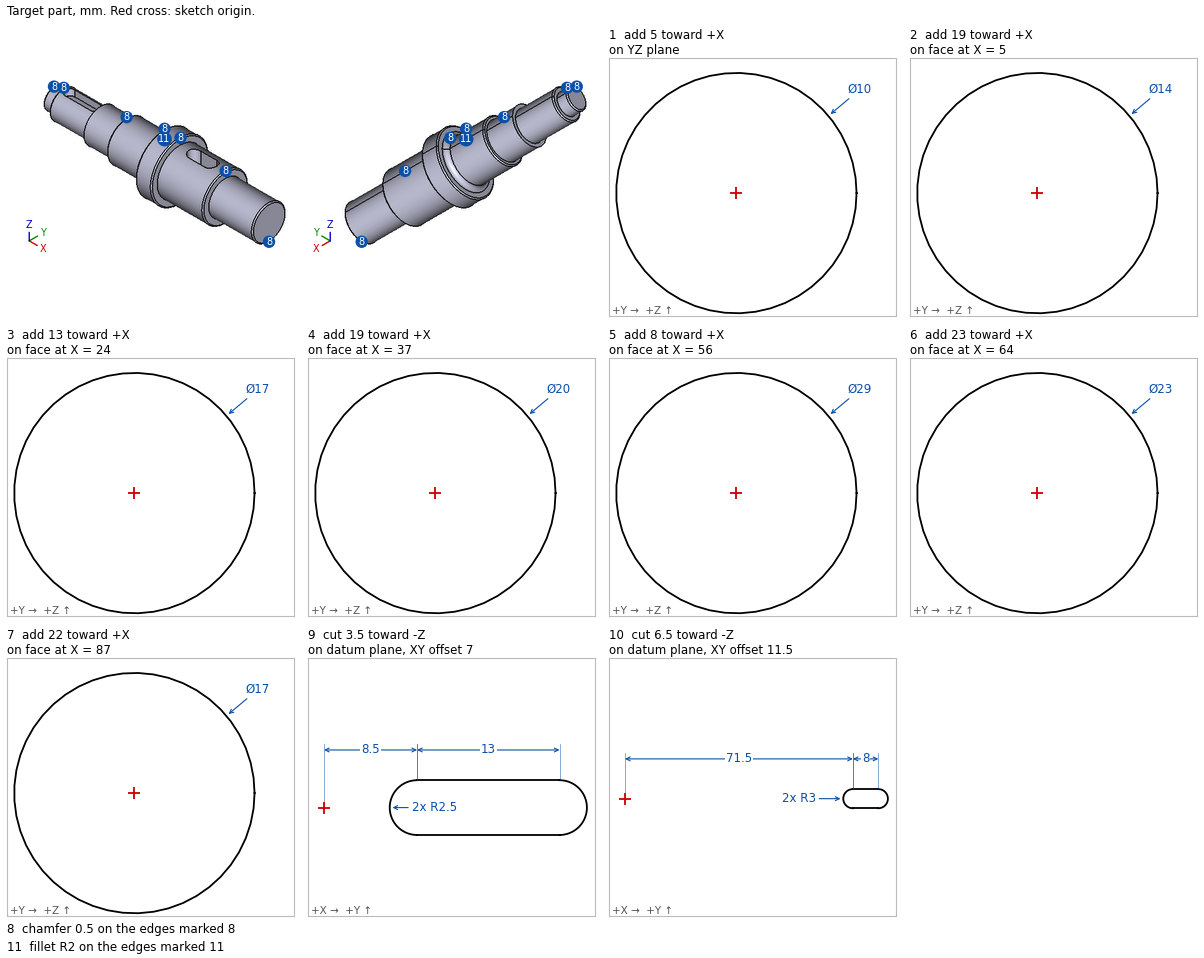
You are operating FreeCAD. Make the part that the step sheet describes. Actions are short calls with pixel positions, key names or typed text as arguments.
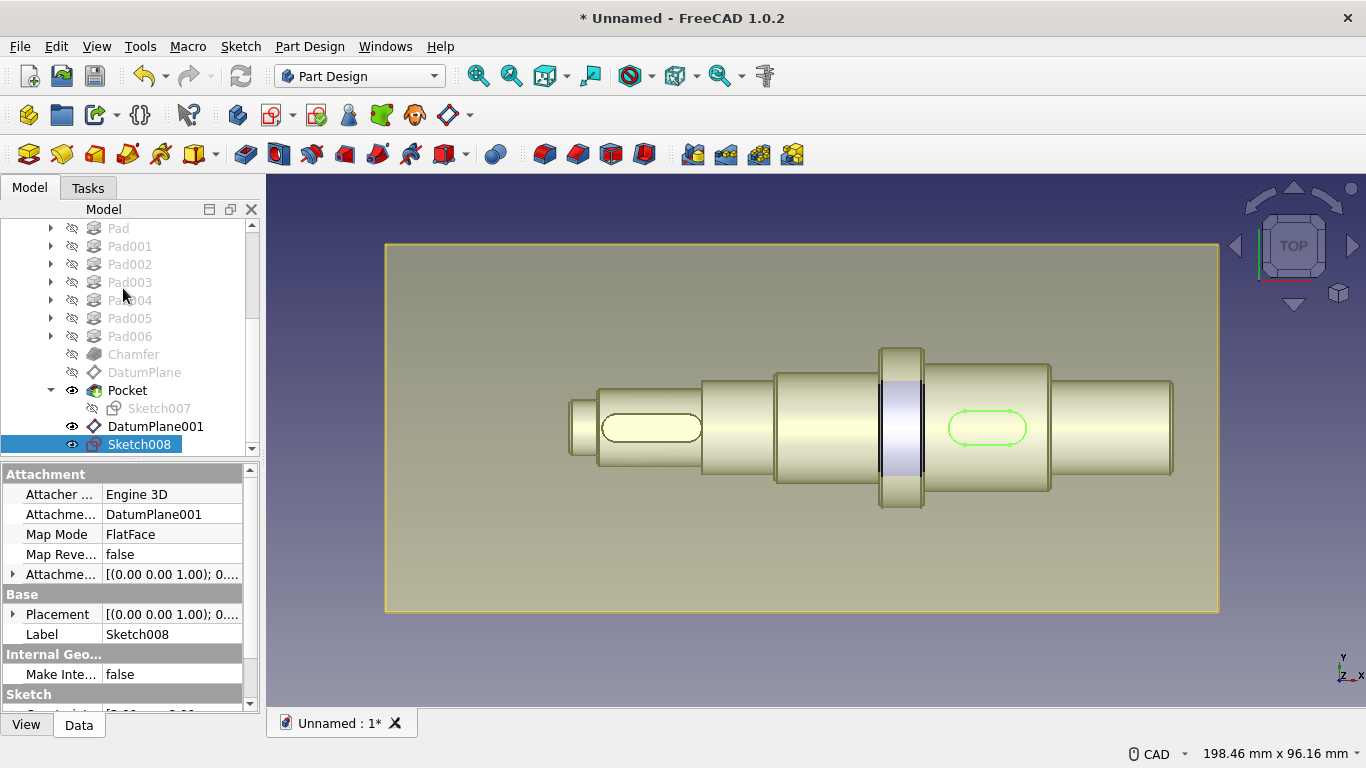
click(246, 154)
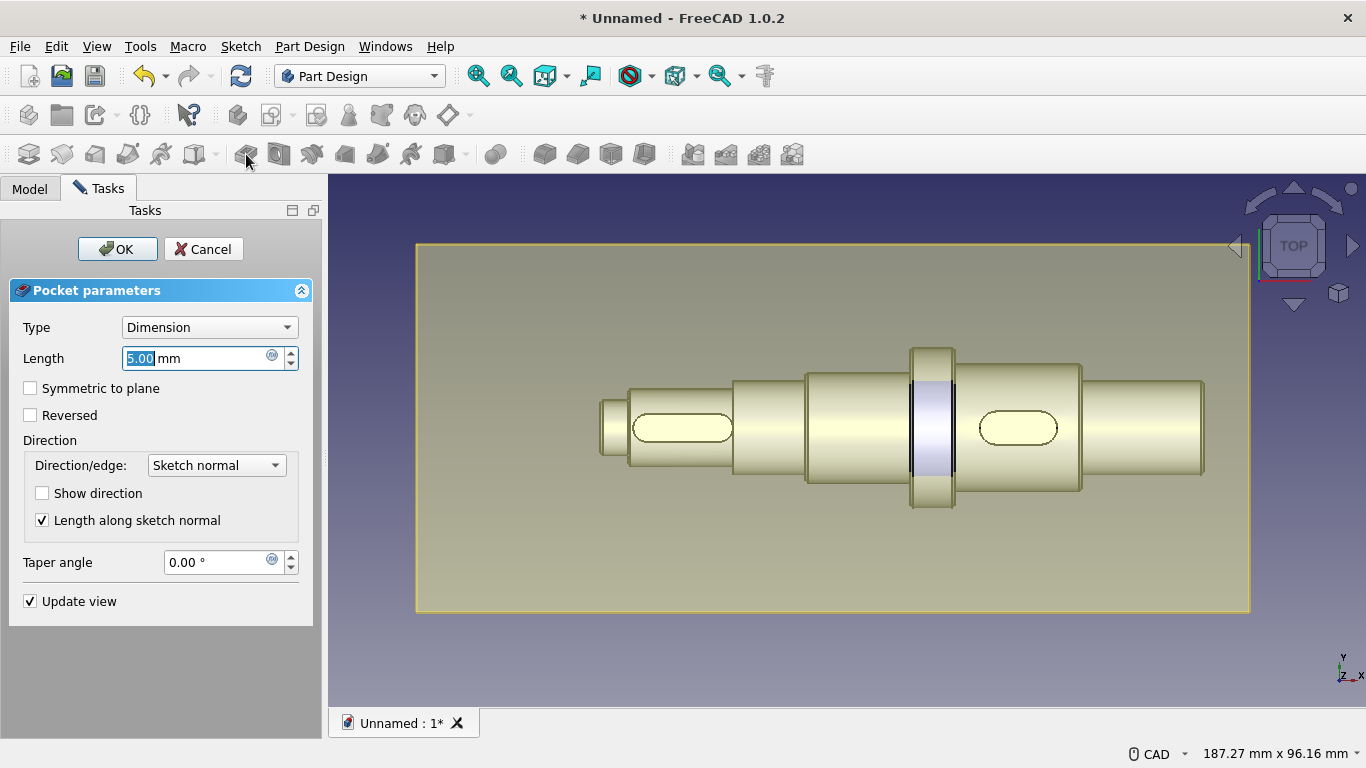
text(6.5)
key(Tab)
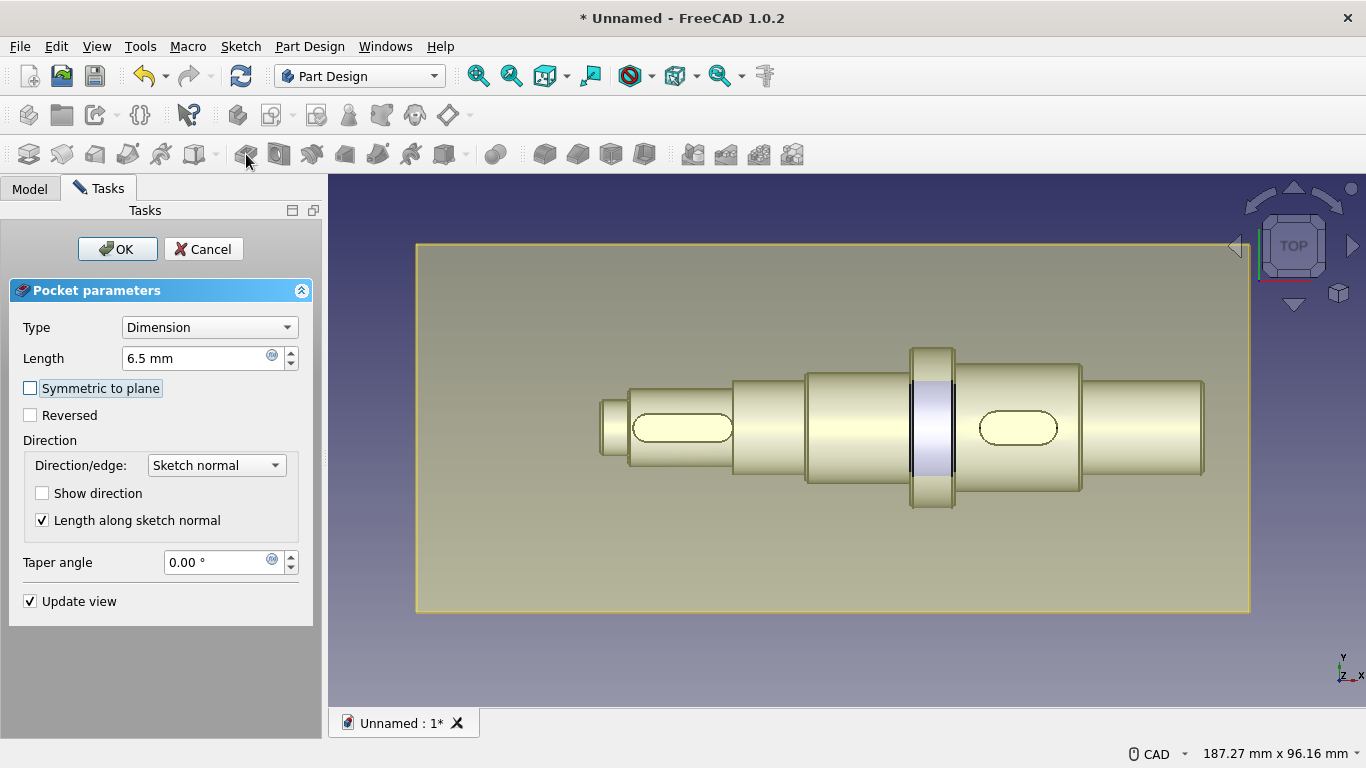
click(118, 249)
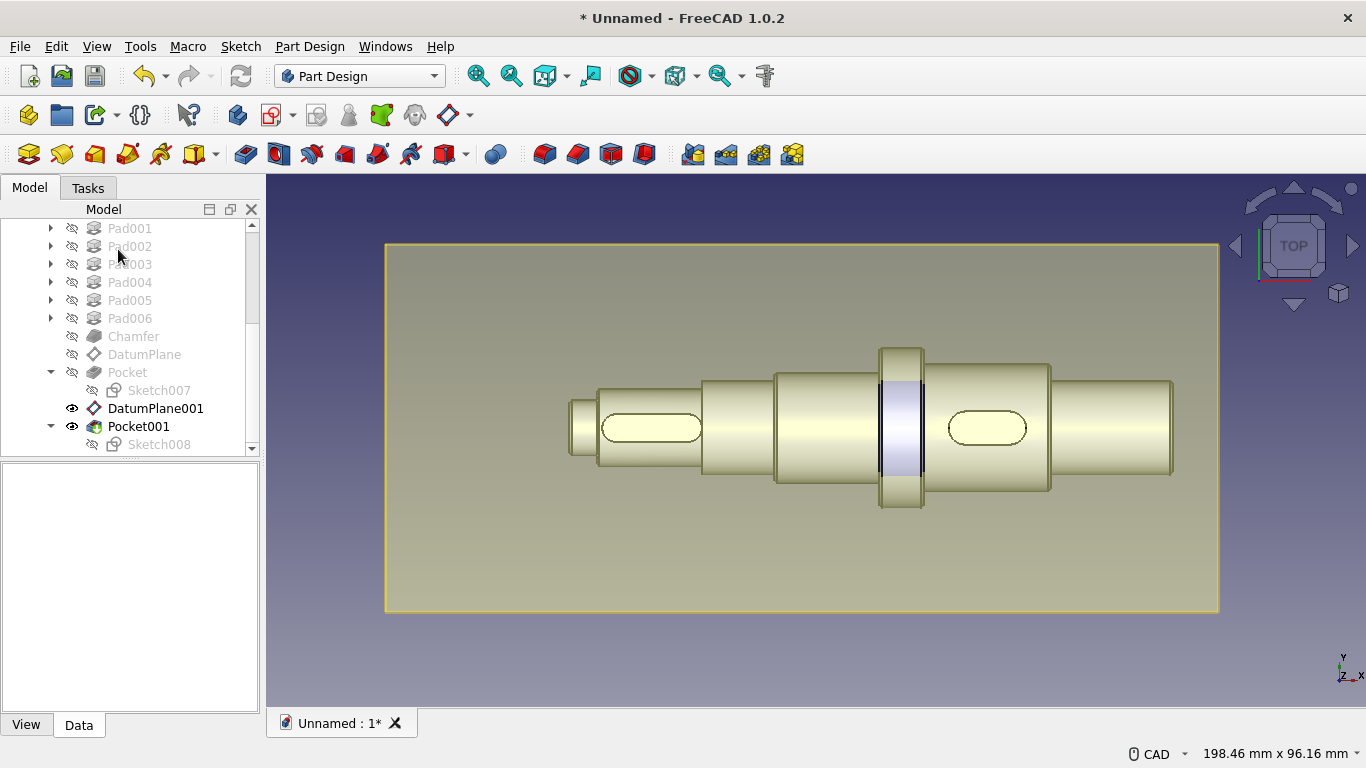
click(117, 408)
key(space)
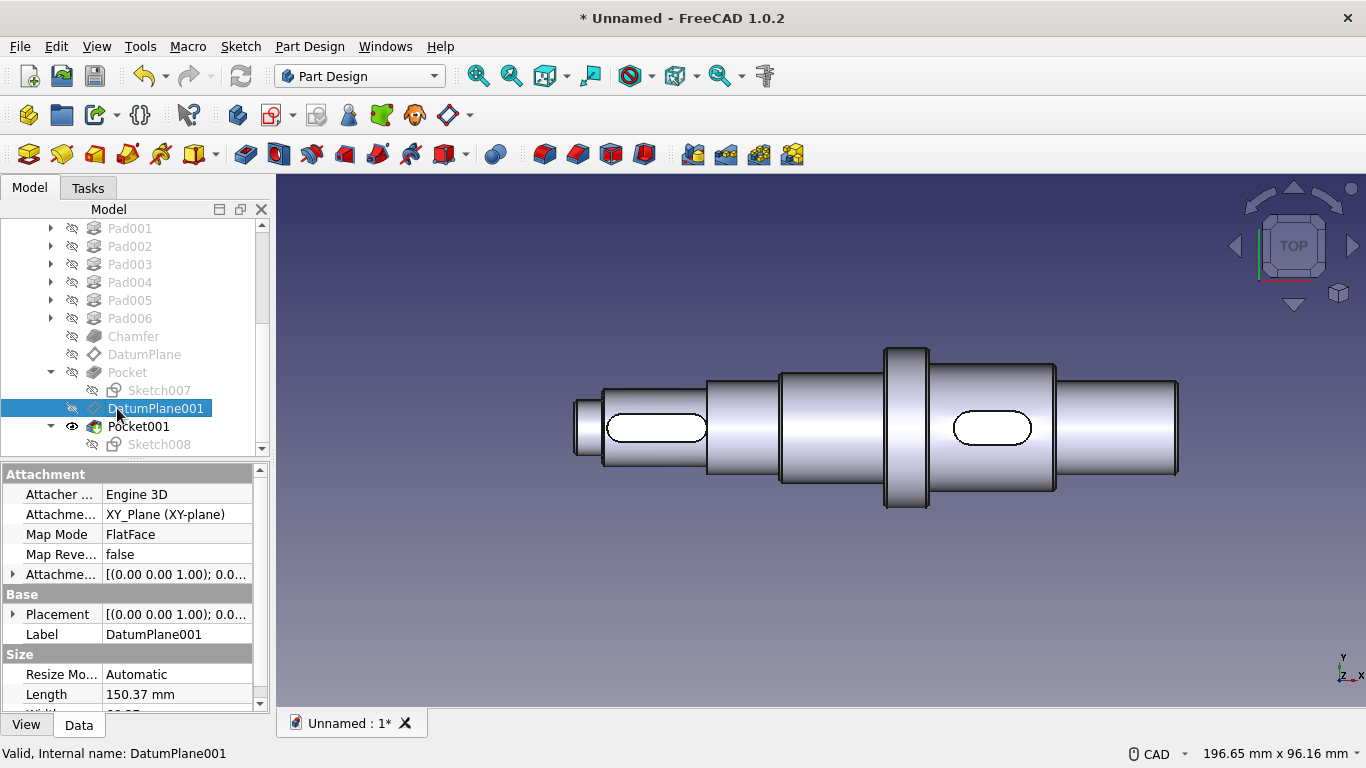
key(0)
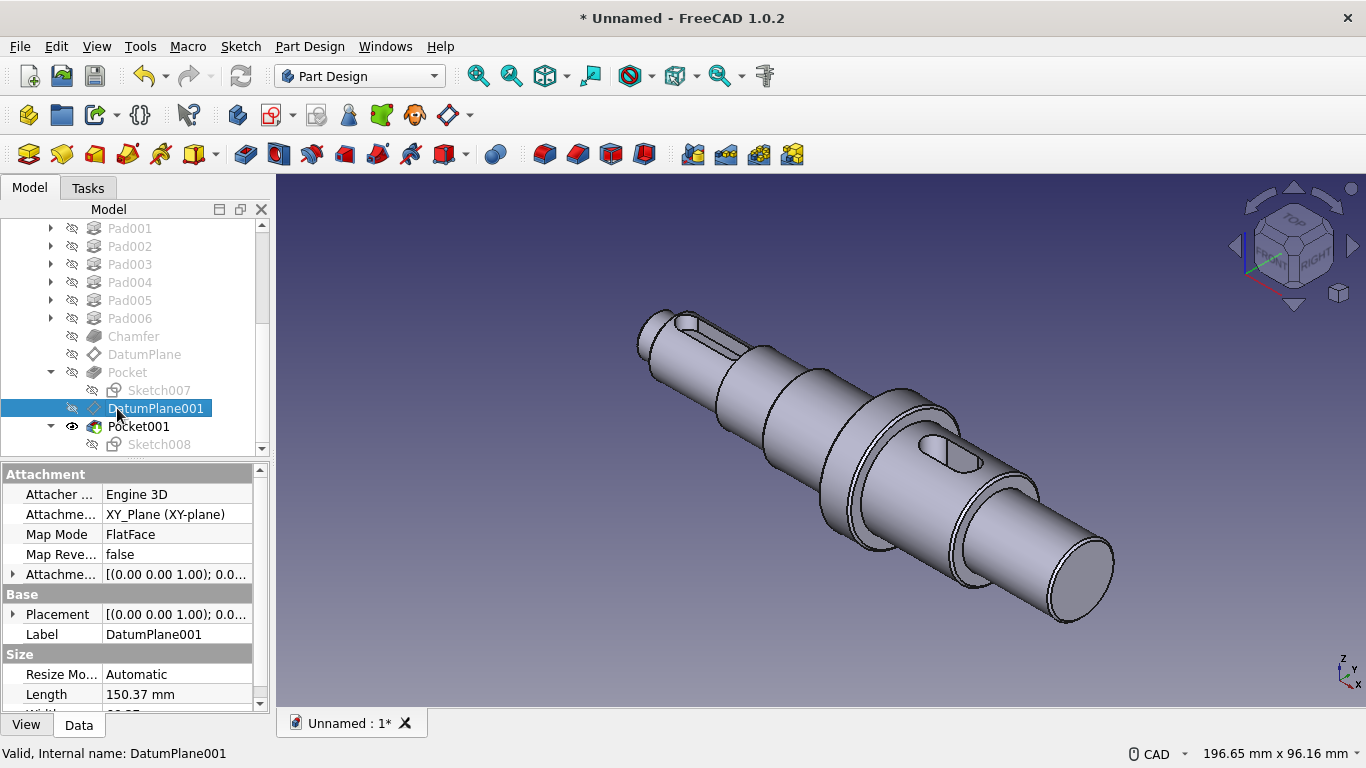
key(2)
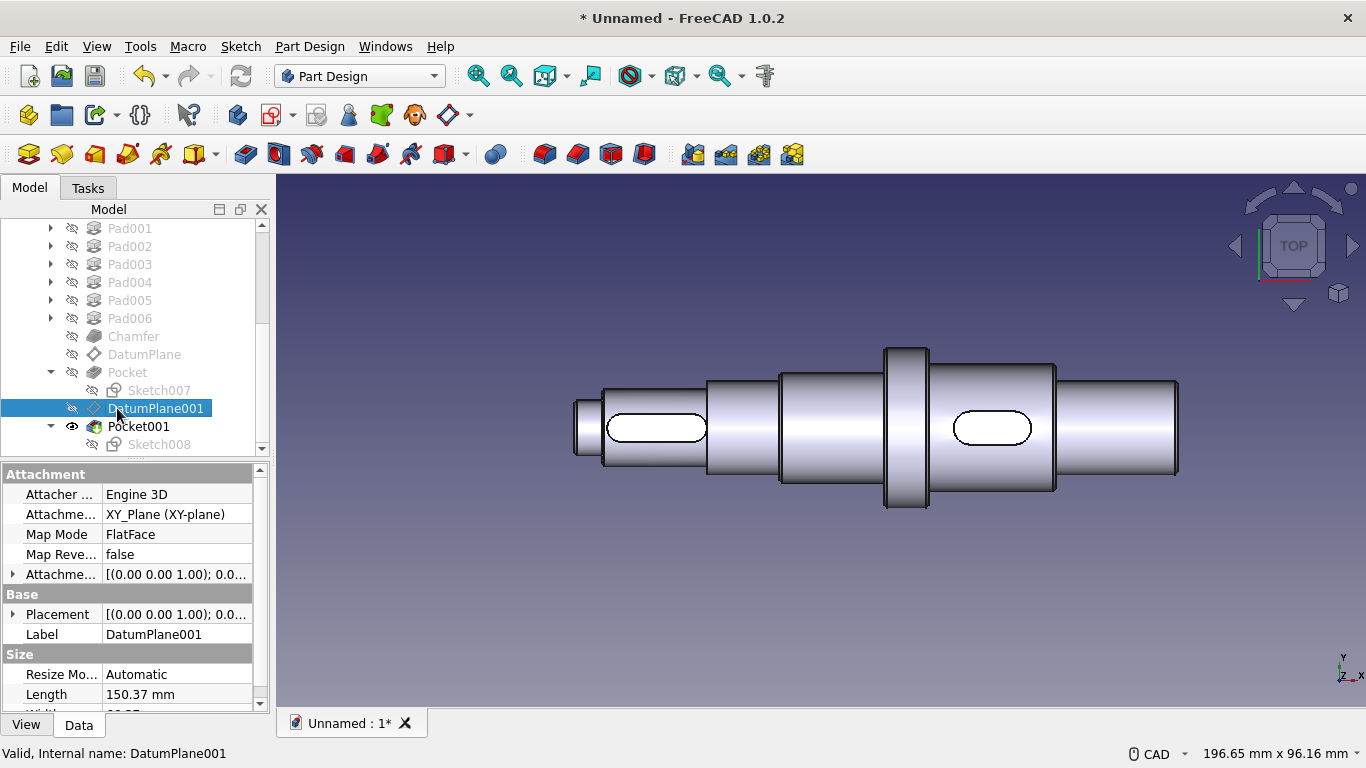
key(1)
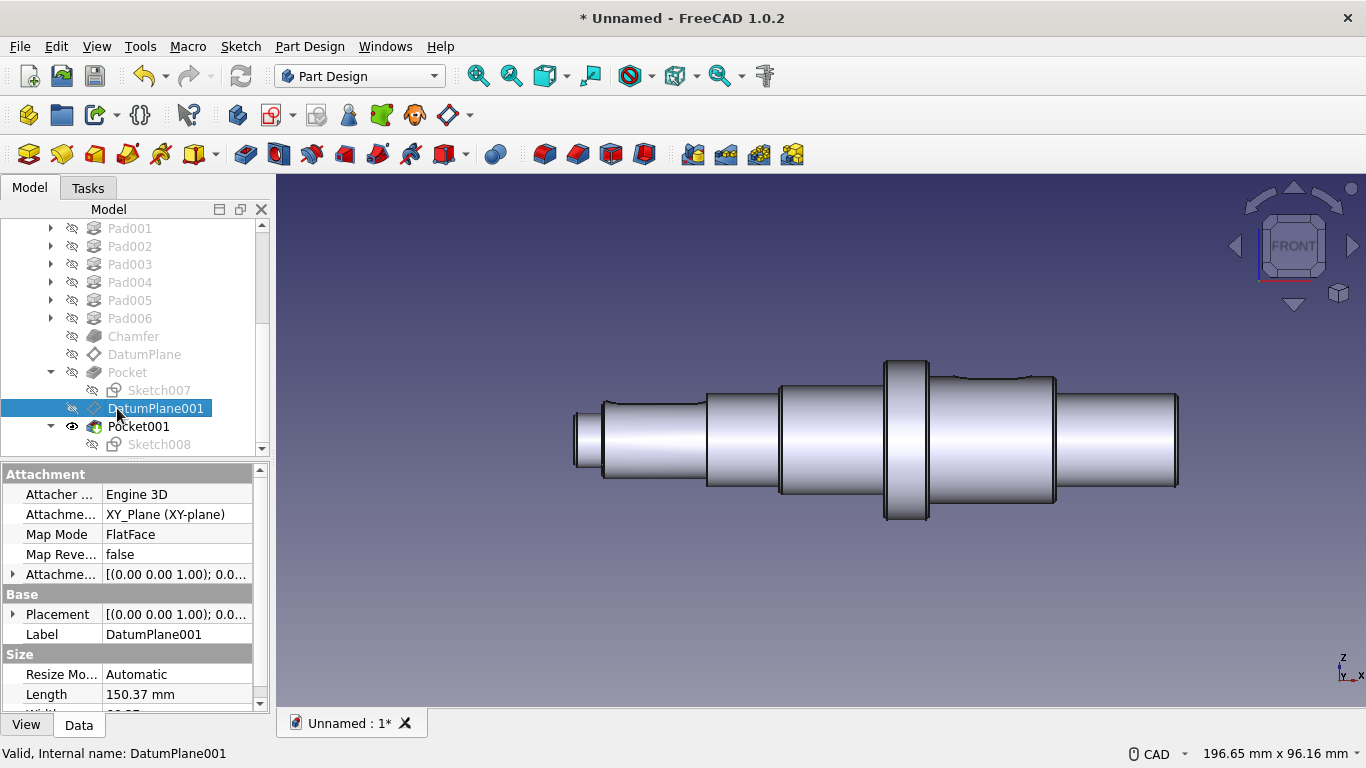
key(3)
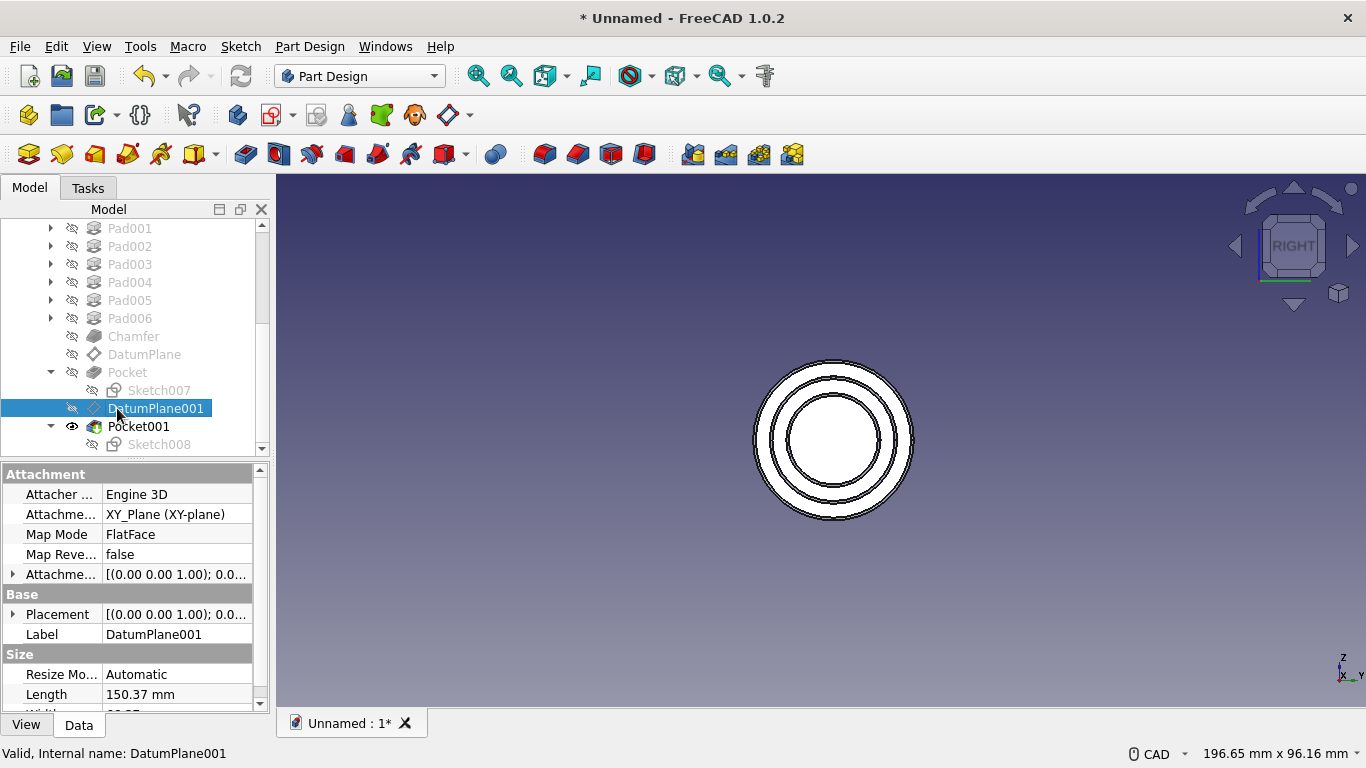
click(479, 76)